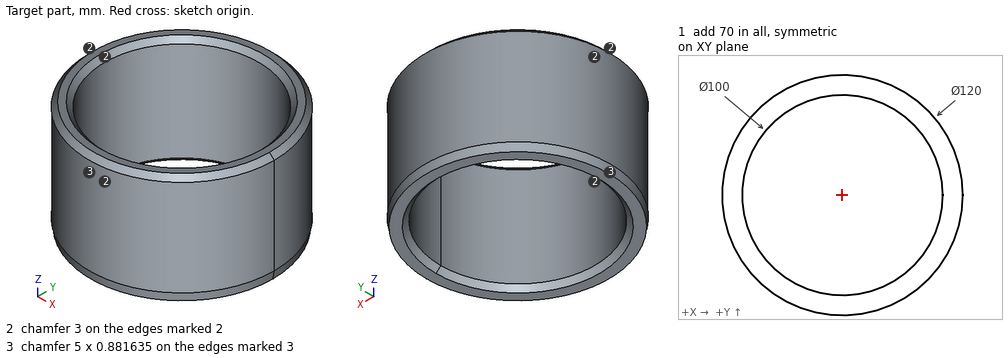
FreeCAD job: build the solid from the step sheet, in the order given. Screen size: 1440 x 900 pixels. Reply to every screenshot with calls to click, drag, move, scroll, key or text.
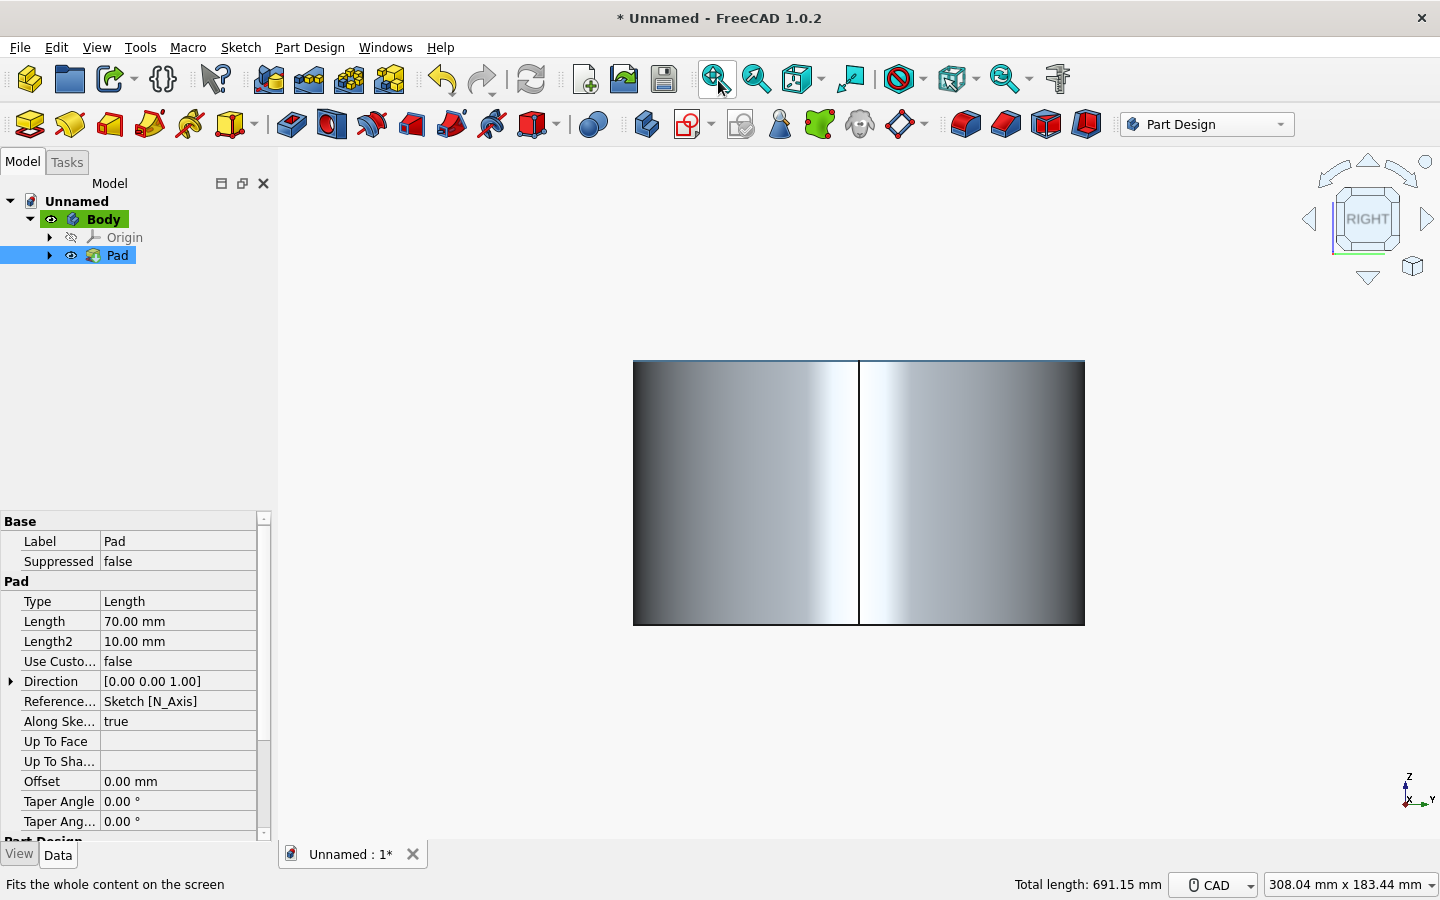
key(5)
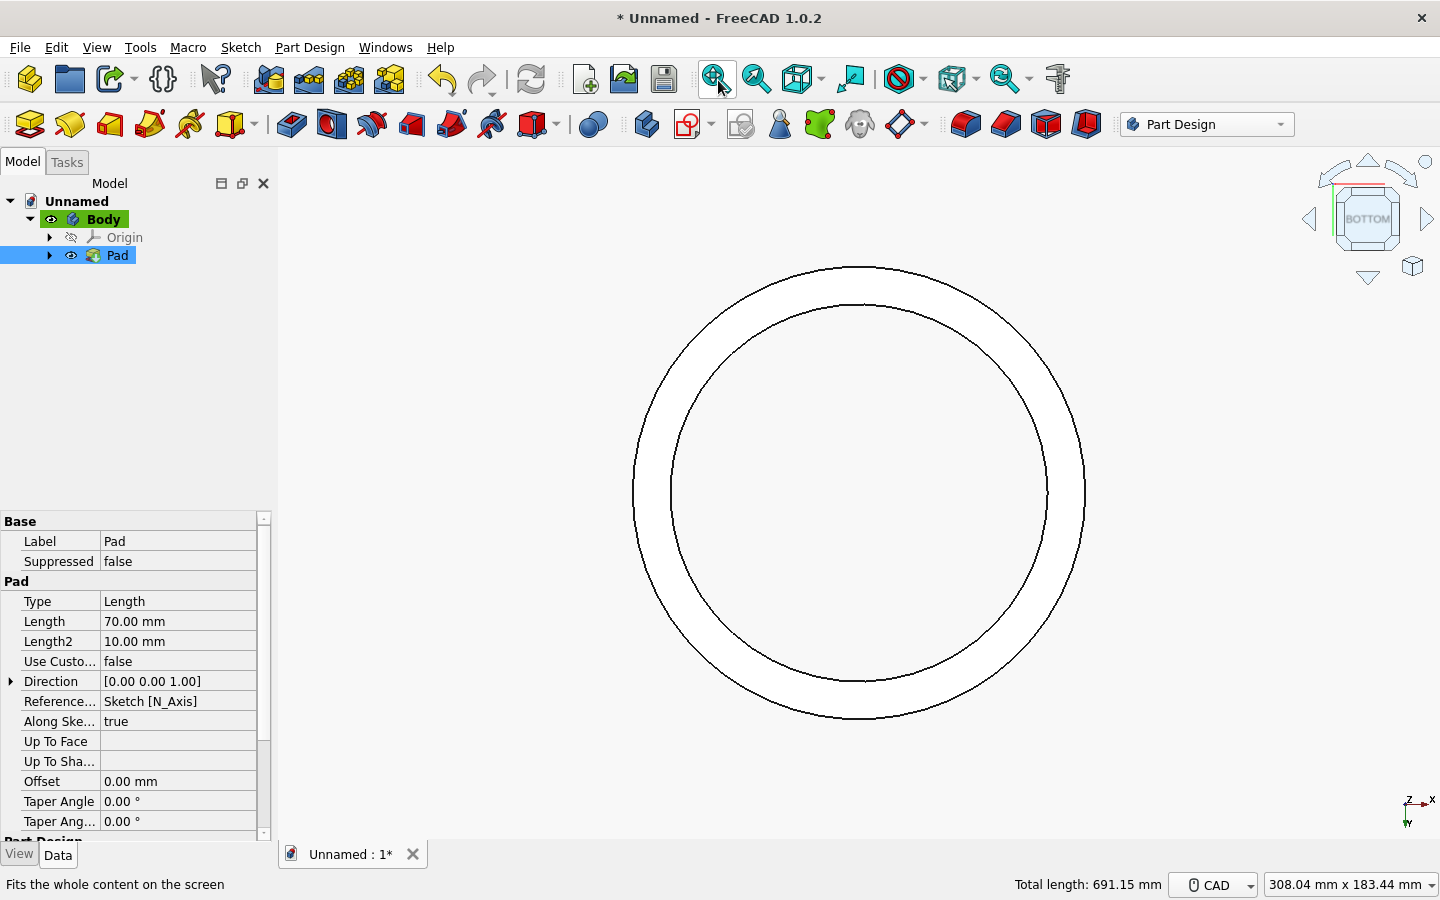
click(670, 492, ctrl)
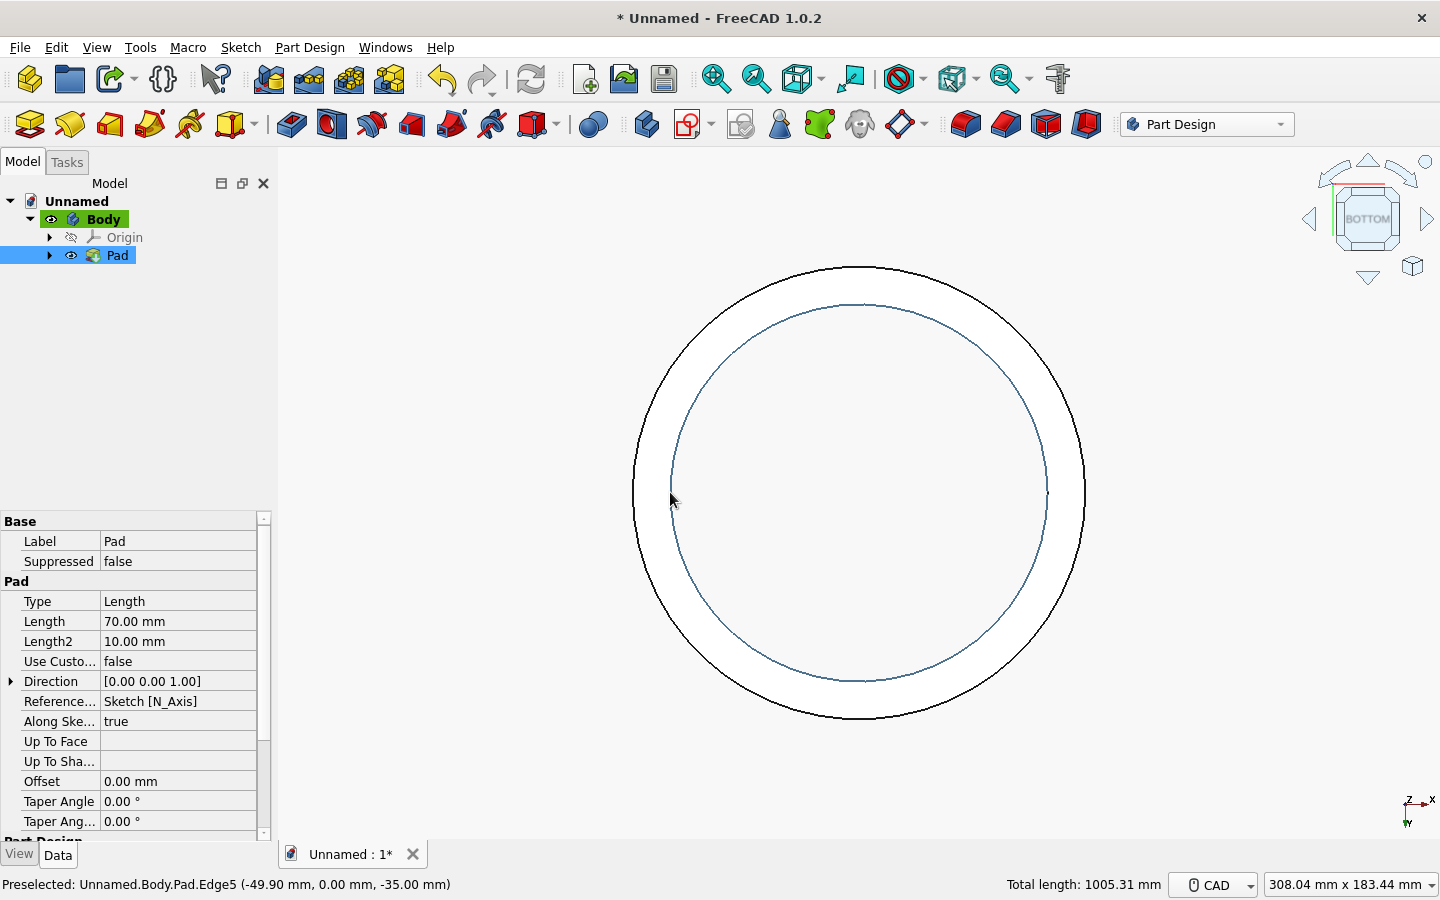
click(1006, 124)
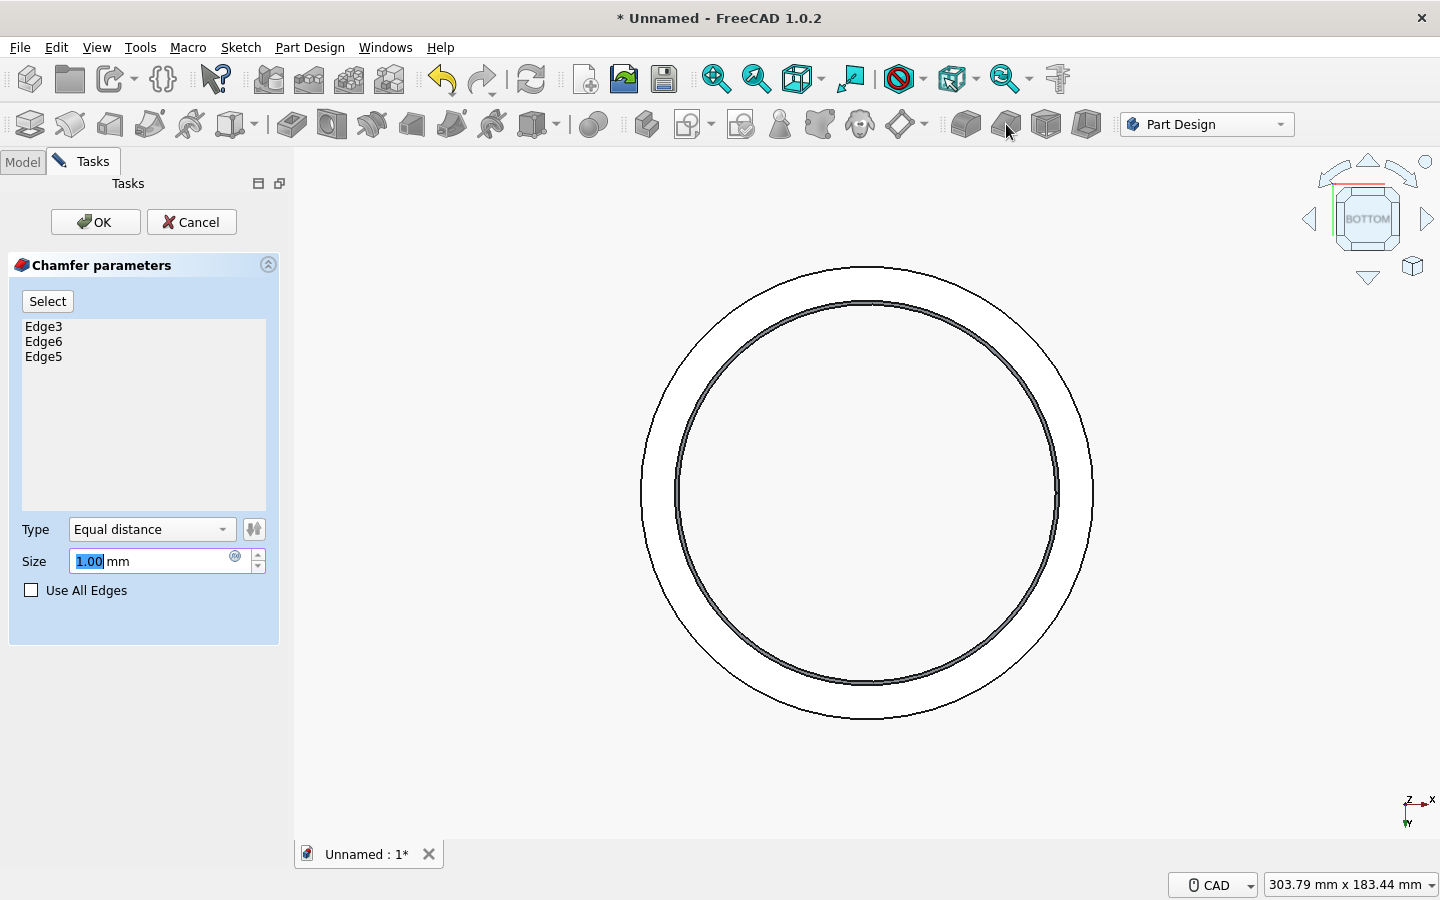
text(3)
key(Tab)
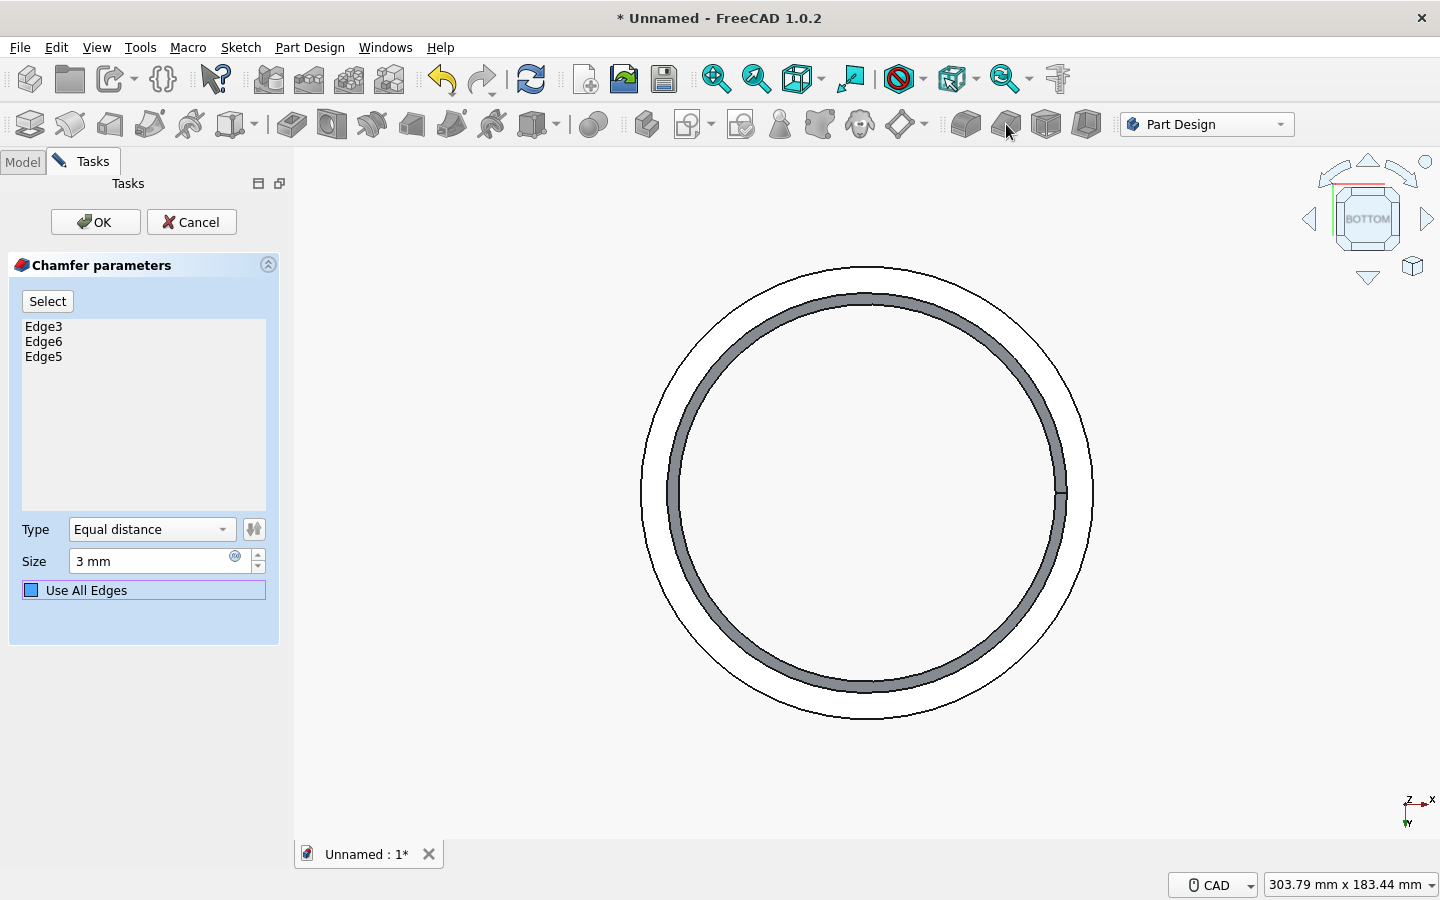
click(96, 222)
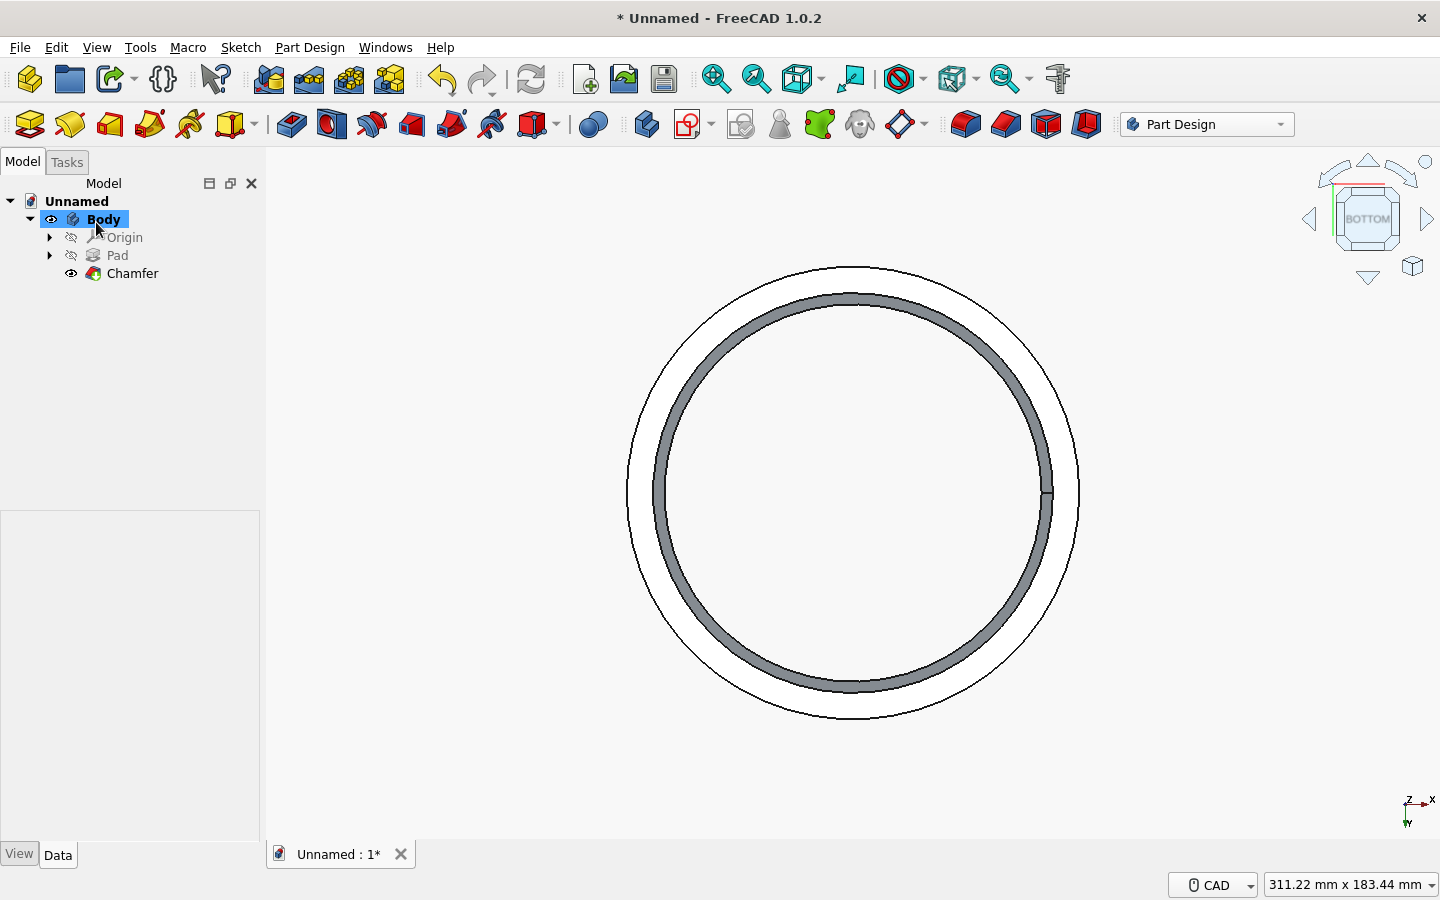
click(627, 492)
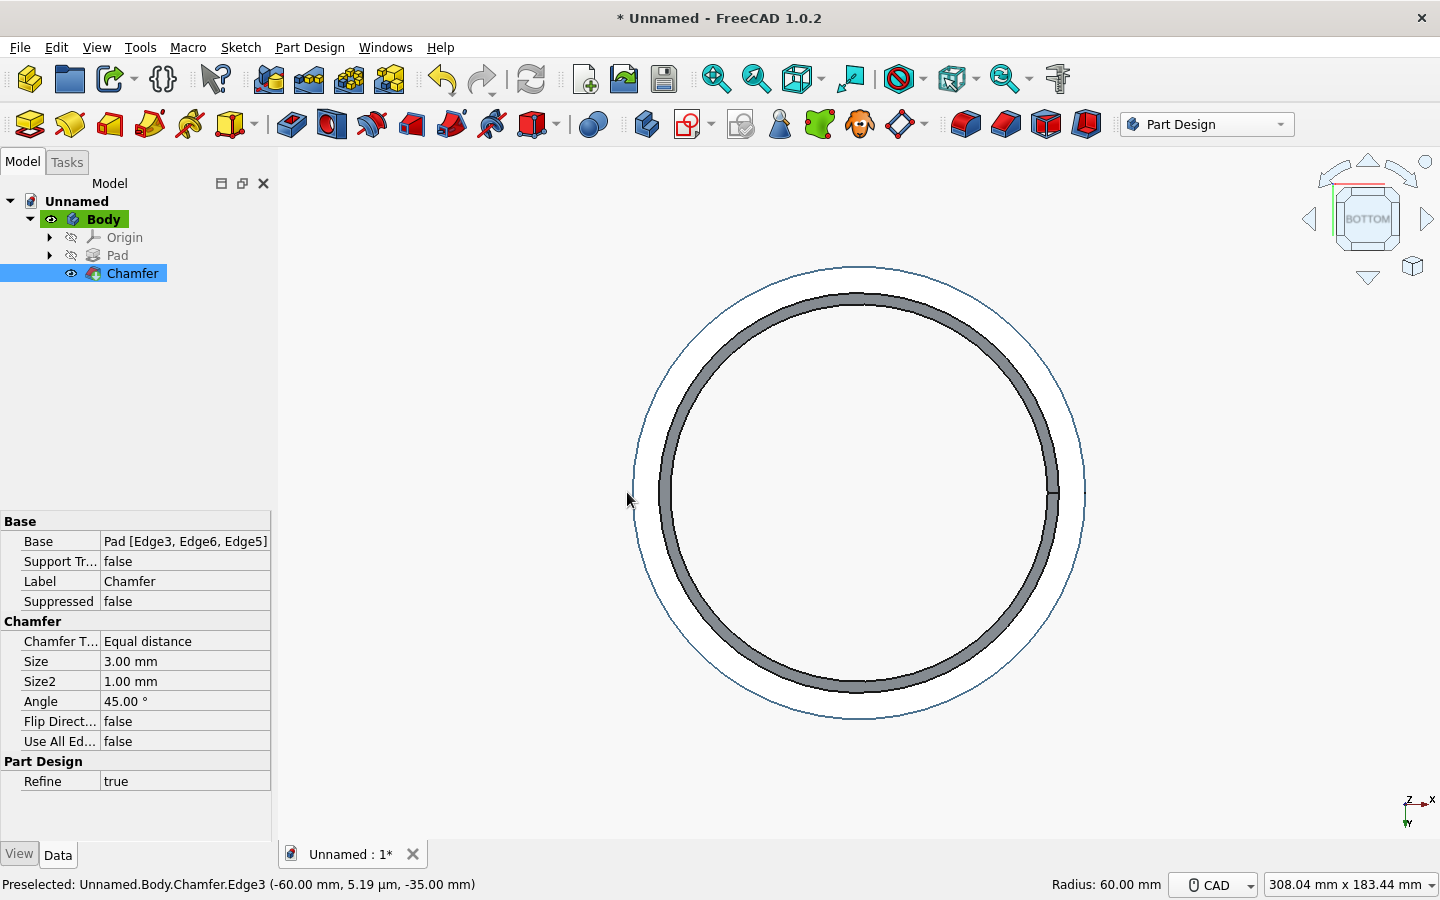
click(1006, 124)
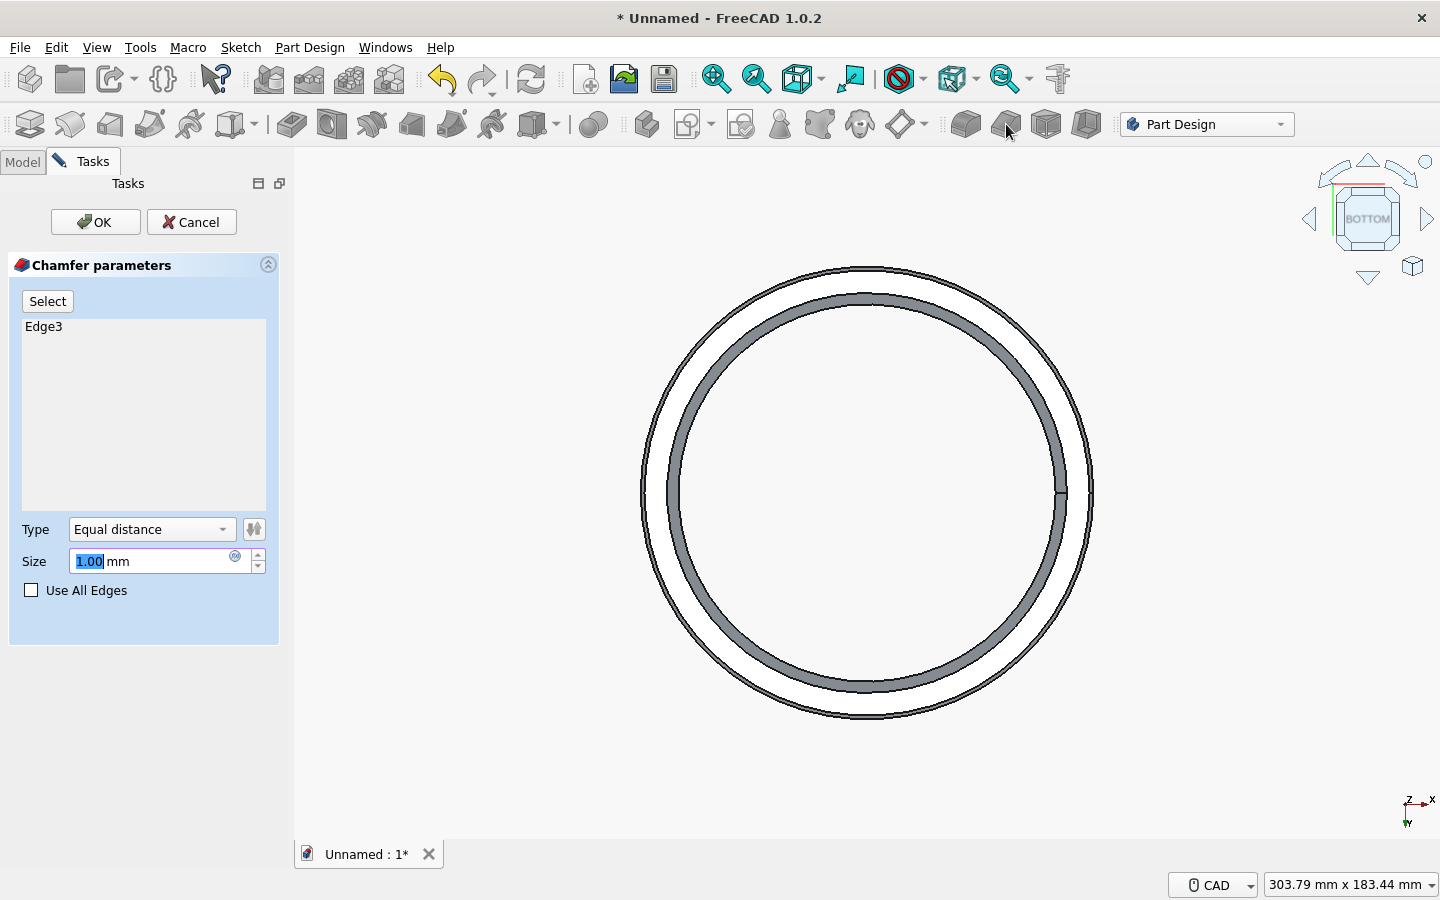
text(5)
key(Tab)